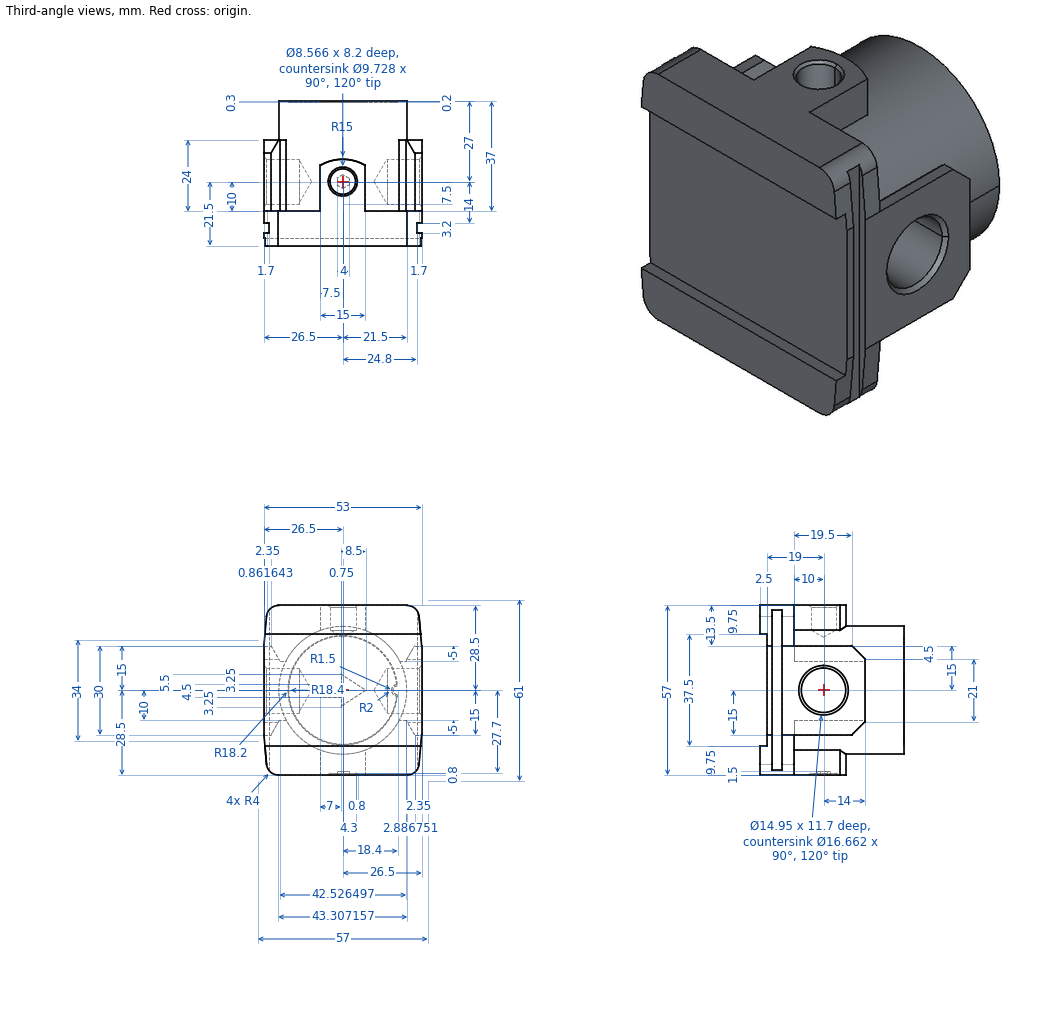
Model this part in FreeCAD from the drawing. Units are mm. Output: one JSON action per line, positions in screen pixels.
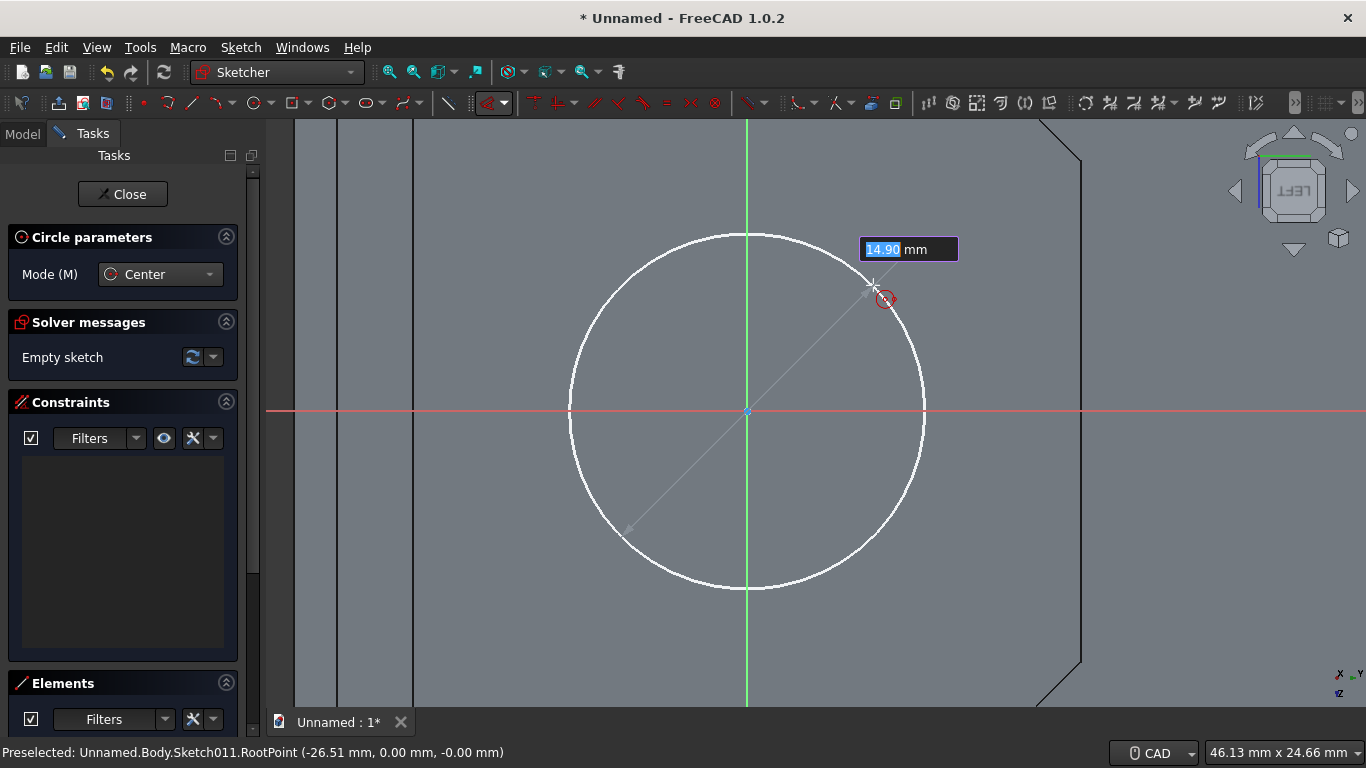
{"action": "type", "text": "14.95"}
{"action": "key", "text": "Return"}
{"action": "key", "text": "Escape"}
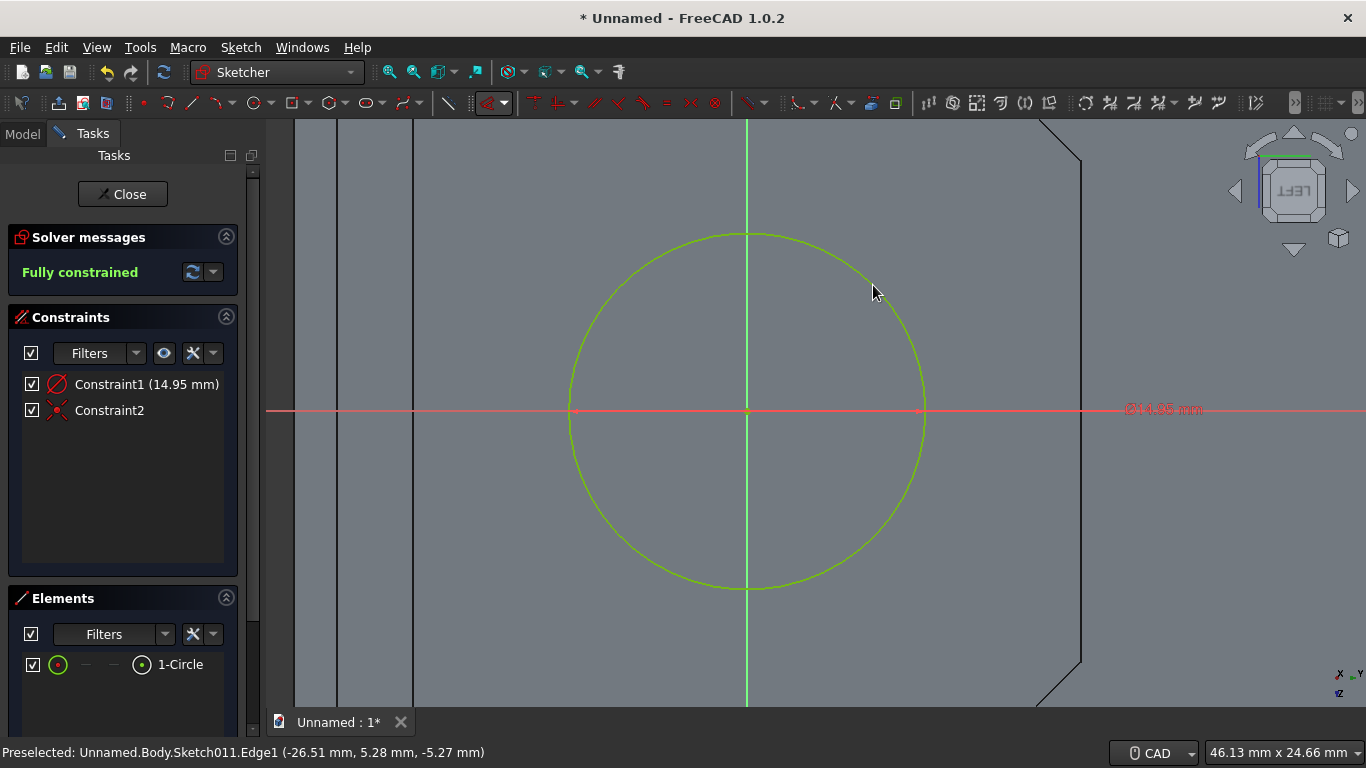
{"action": "left_click", "coordinate": [123, 194]}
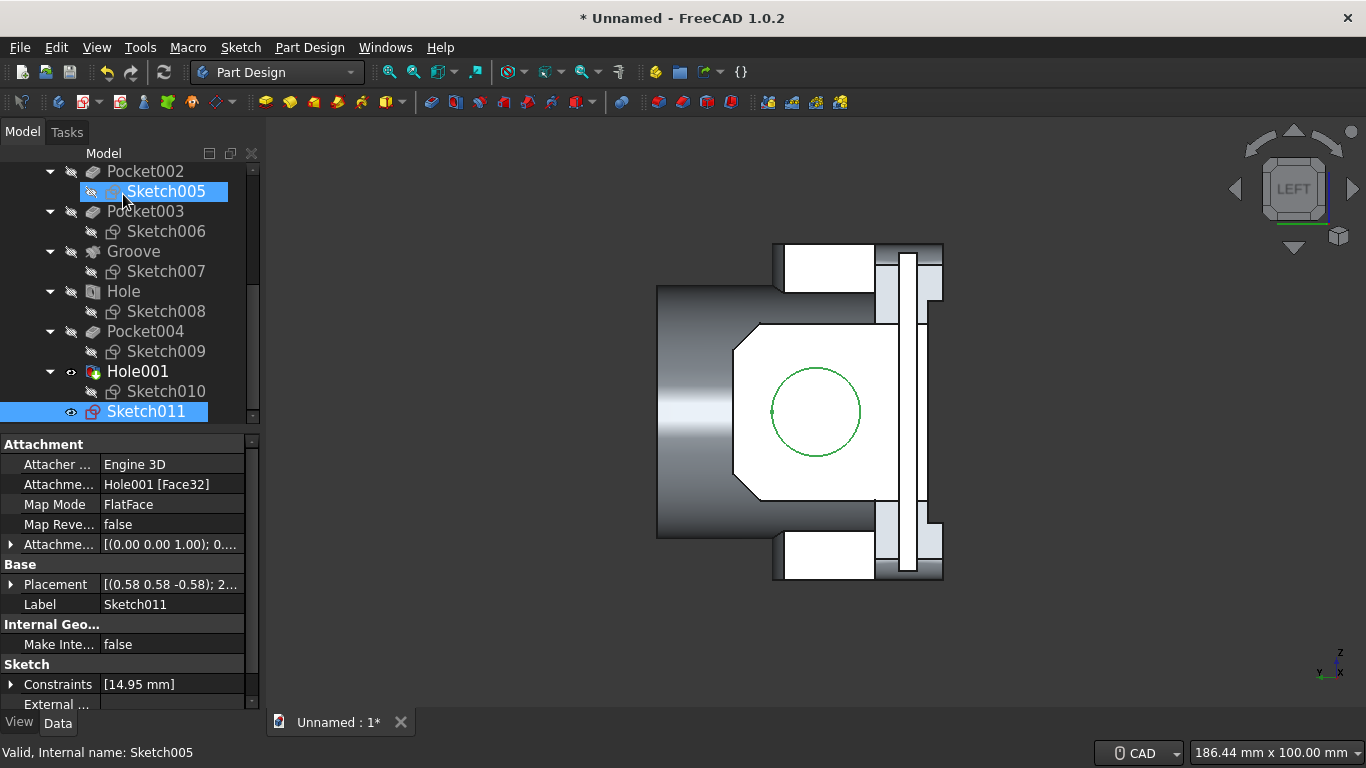
{"action": "left_click", "coordinate": [456, 102]}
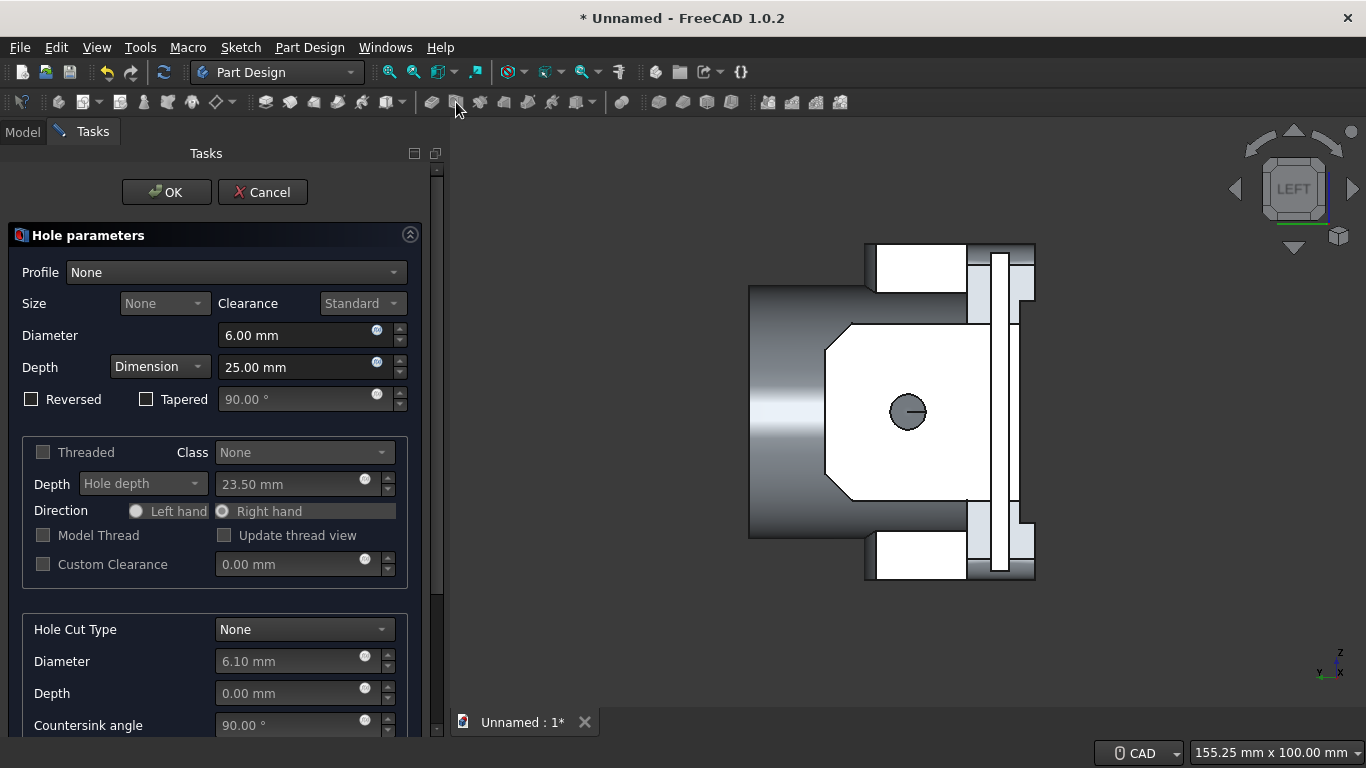
{"action": "triple_click", "coordinate": [305, 335]}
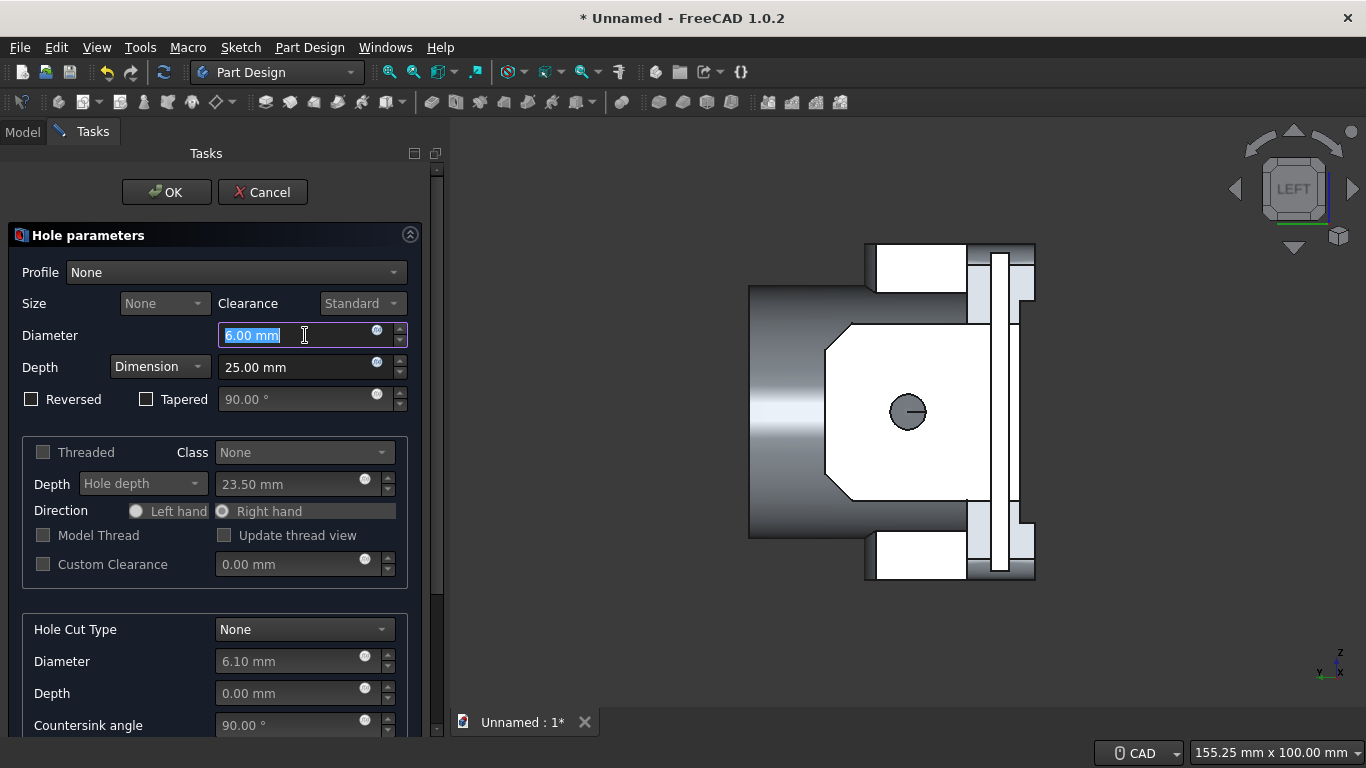
{"action": "type", "text": "14.95"}
{"action": "key", "text": "Tab"}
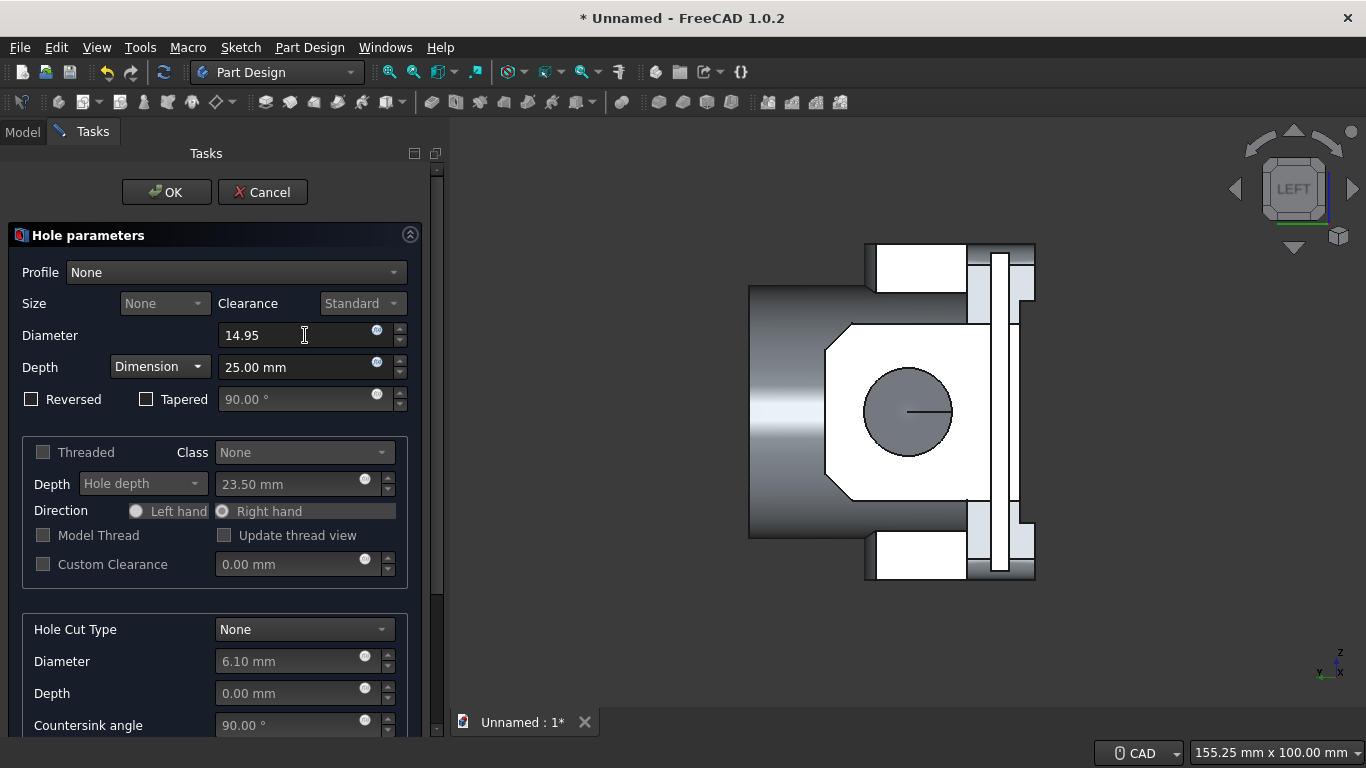
{"action": "triple_click", "coordinate": [305, 367]}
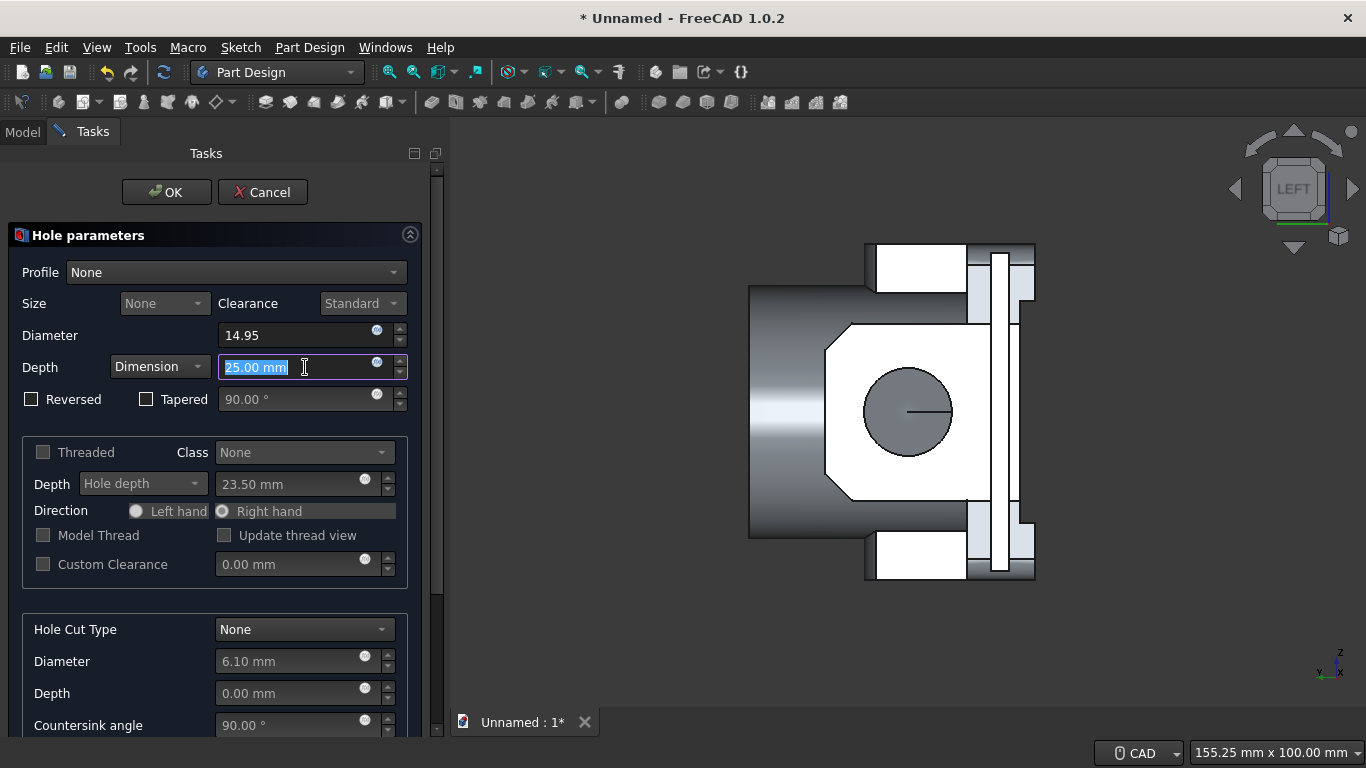
{"action": "type", "text": "11.7"}
{"action": "key", "text": "Tab"}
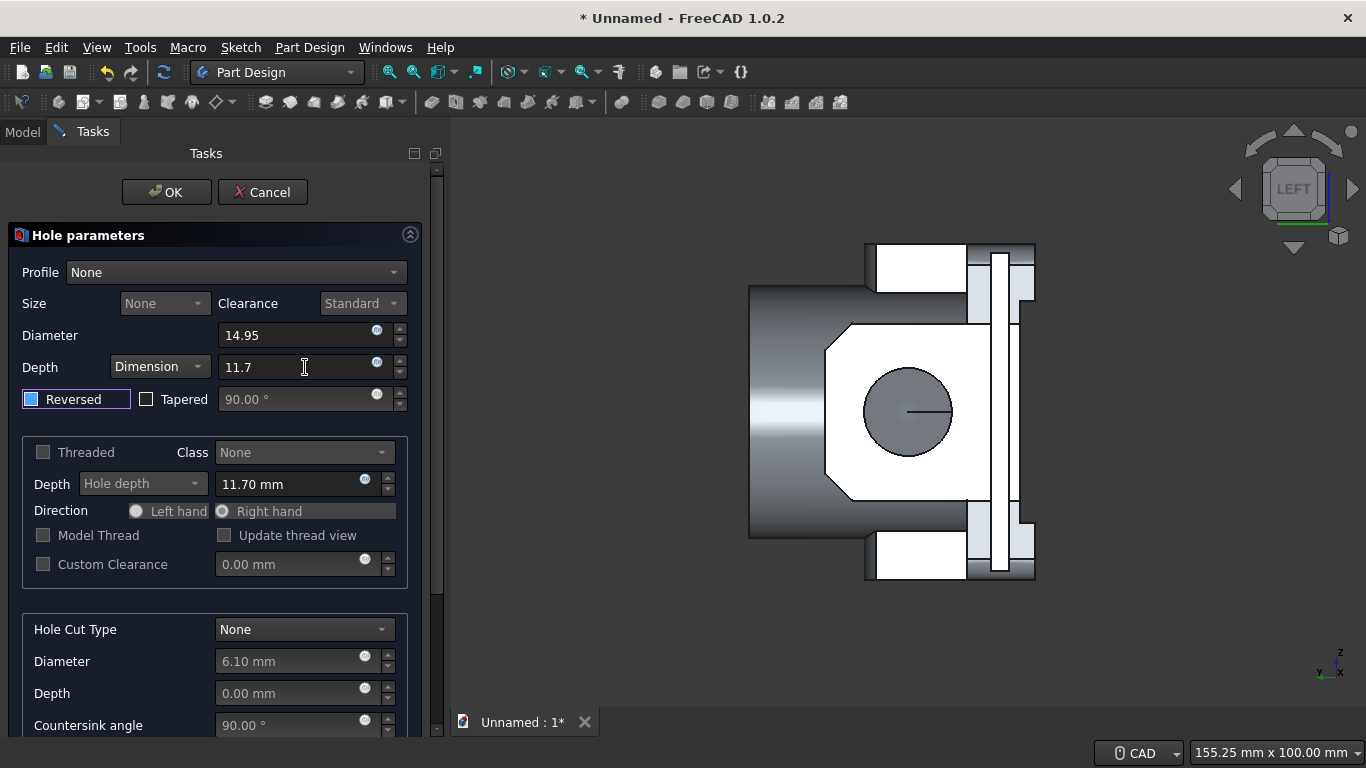
{"action": "left_click", "coordinate": [306, 630]}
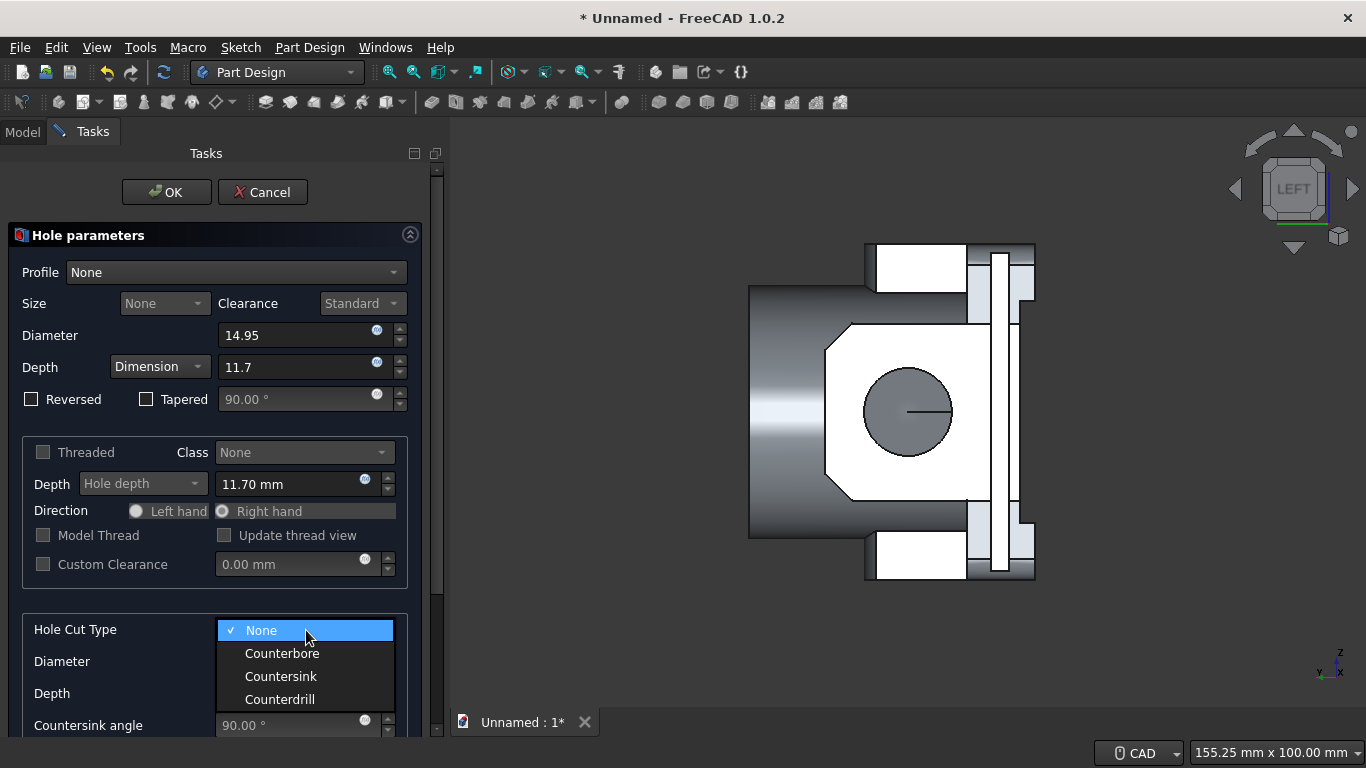
{"action": "left_click", "coordinate": [304, 676]}